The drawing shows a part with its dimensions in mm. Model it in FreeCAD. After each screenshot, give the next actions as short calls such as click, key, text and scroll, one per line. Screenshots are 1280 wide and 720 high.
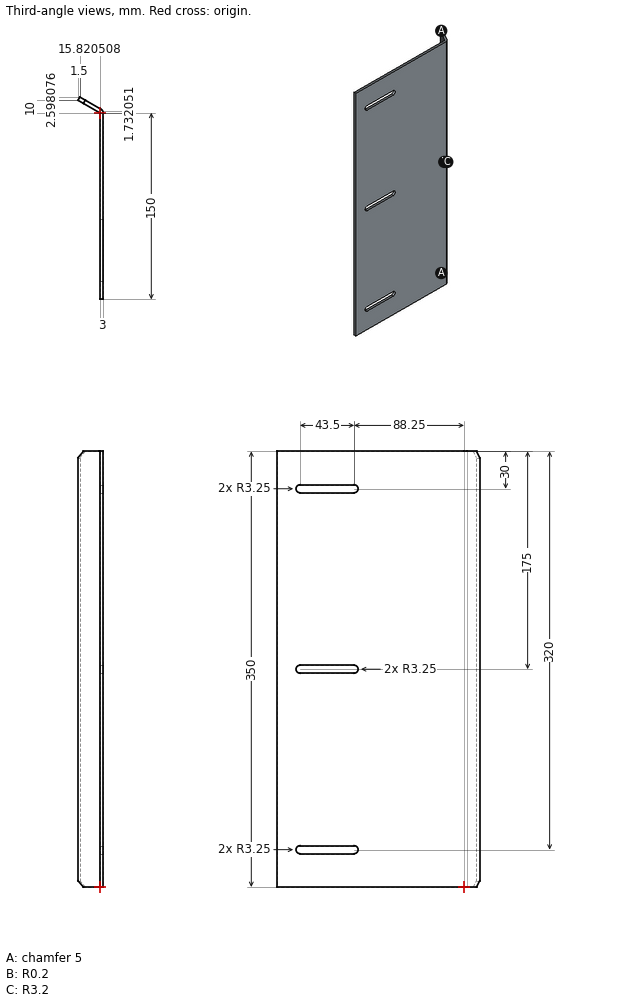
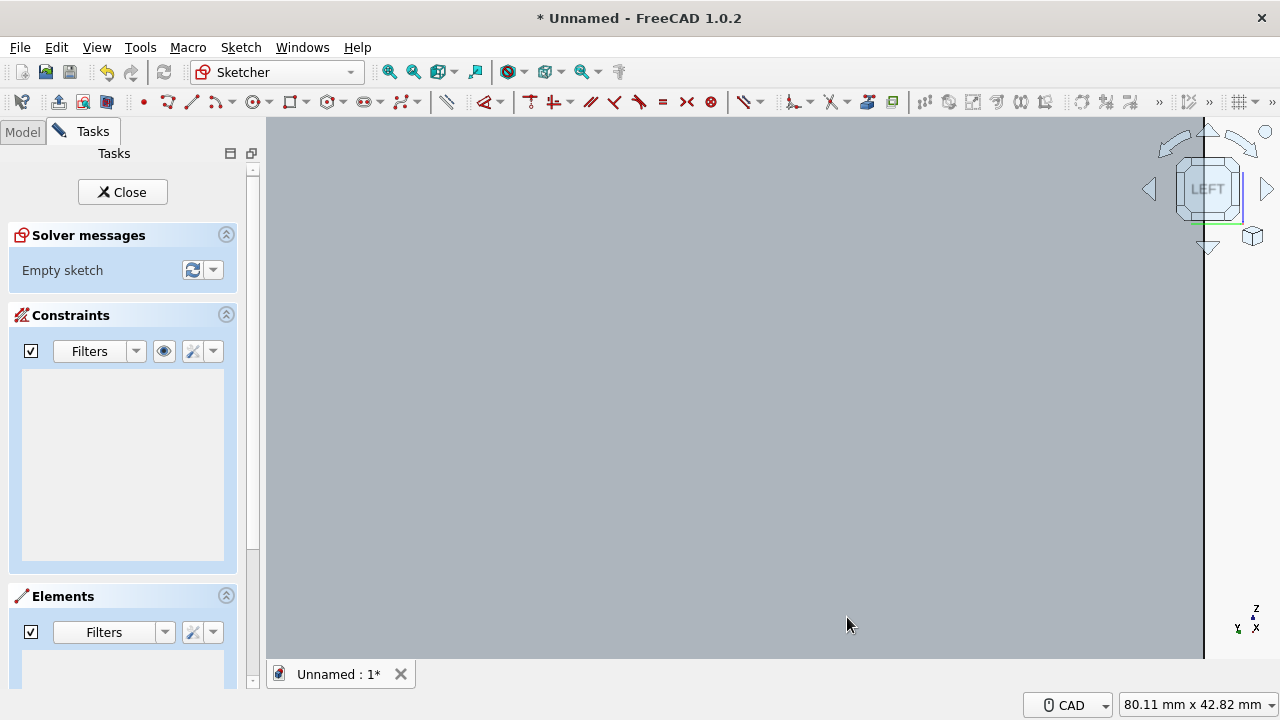
key(g)
key(s)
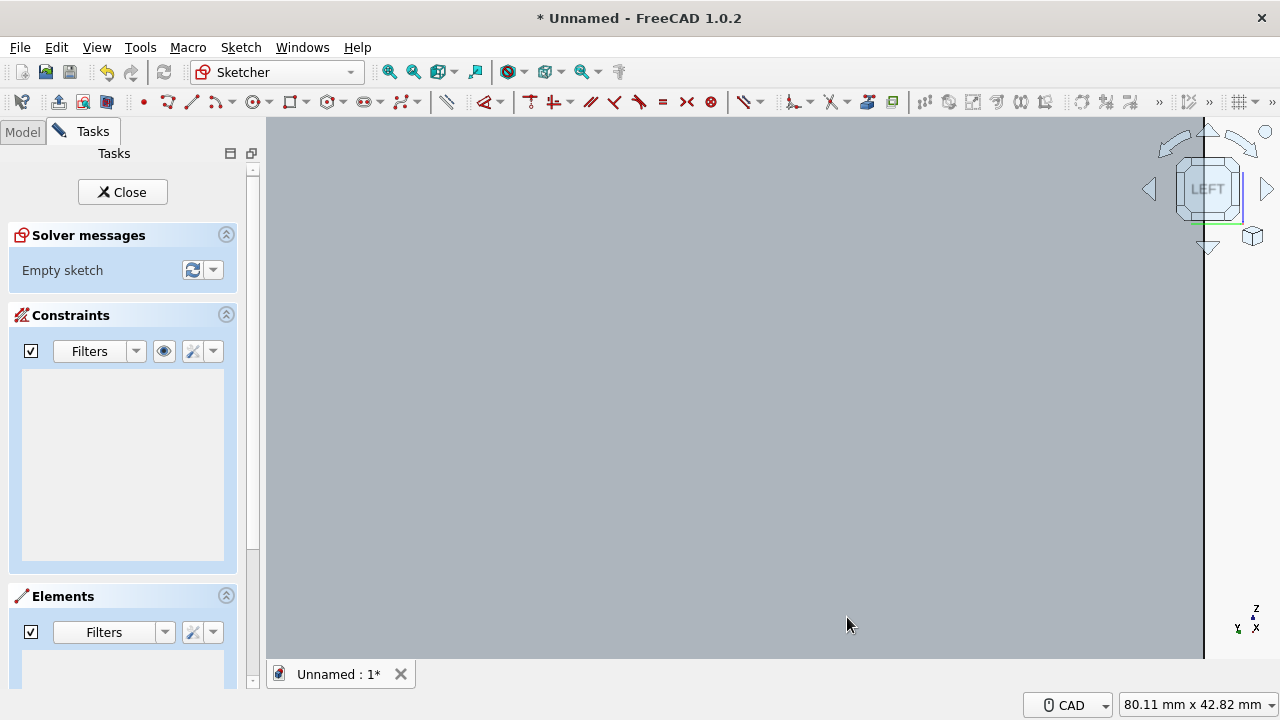
click(422, 378)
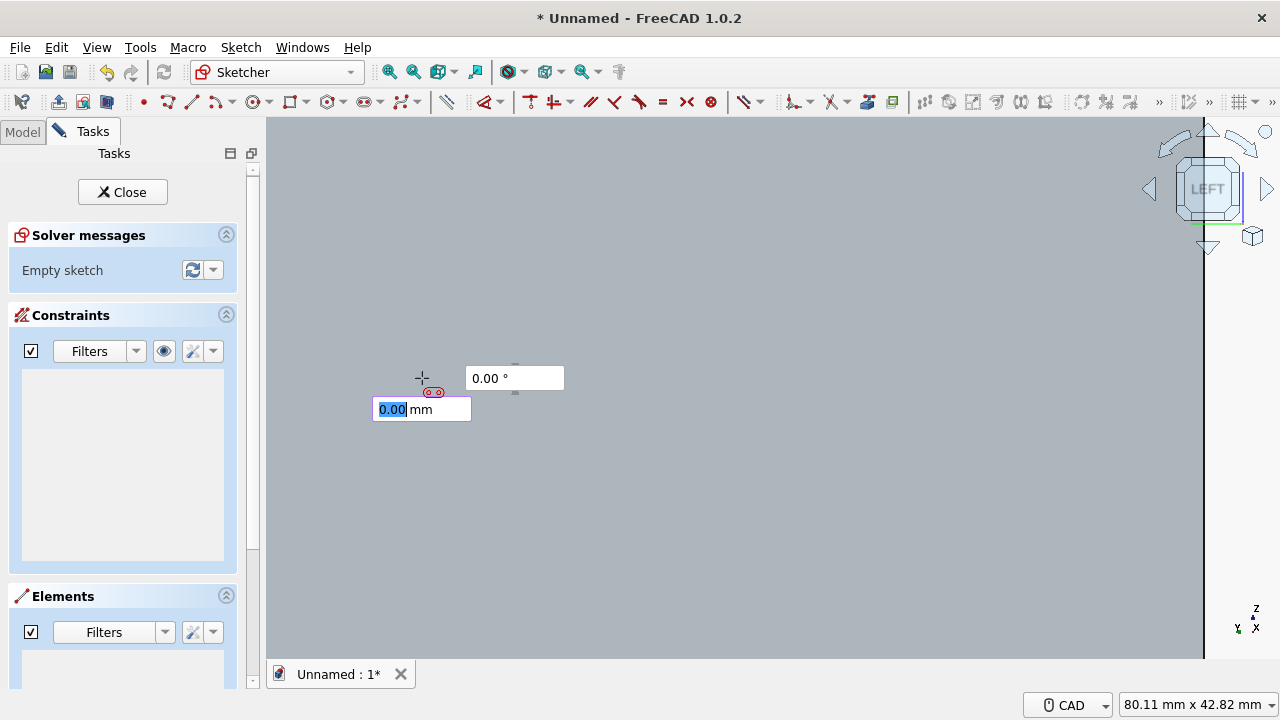
click(973, 378)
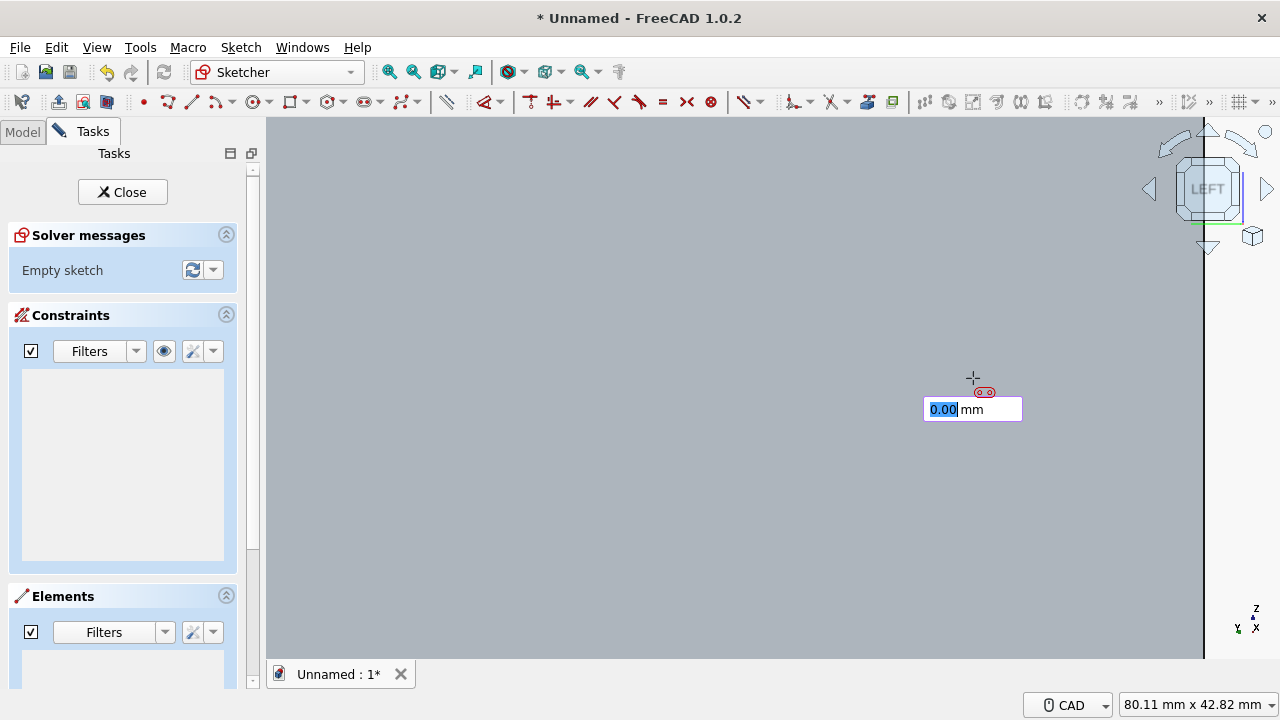
click(697, 419)
key(Escape)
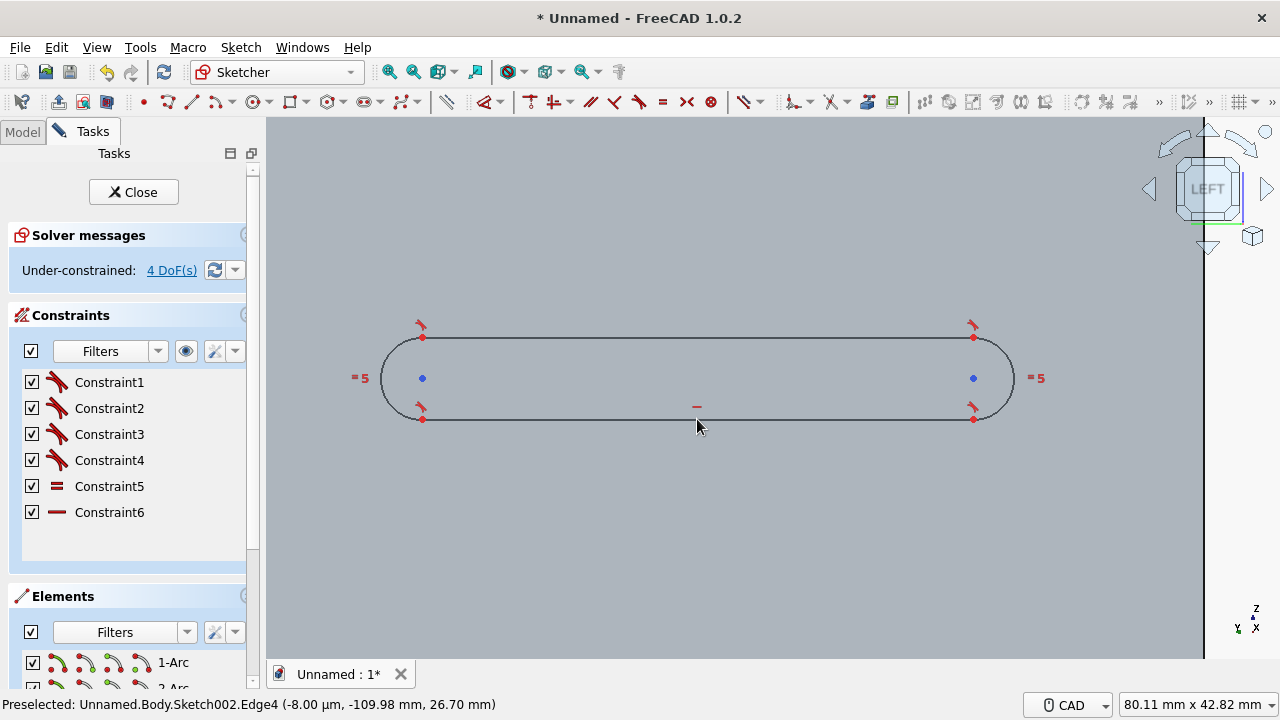
click(484, 102)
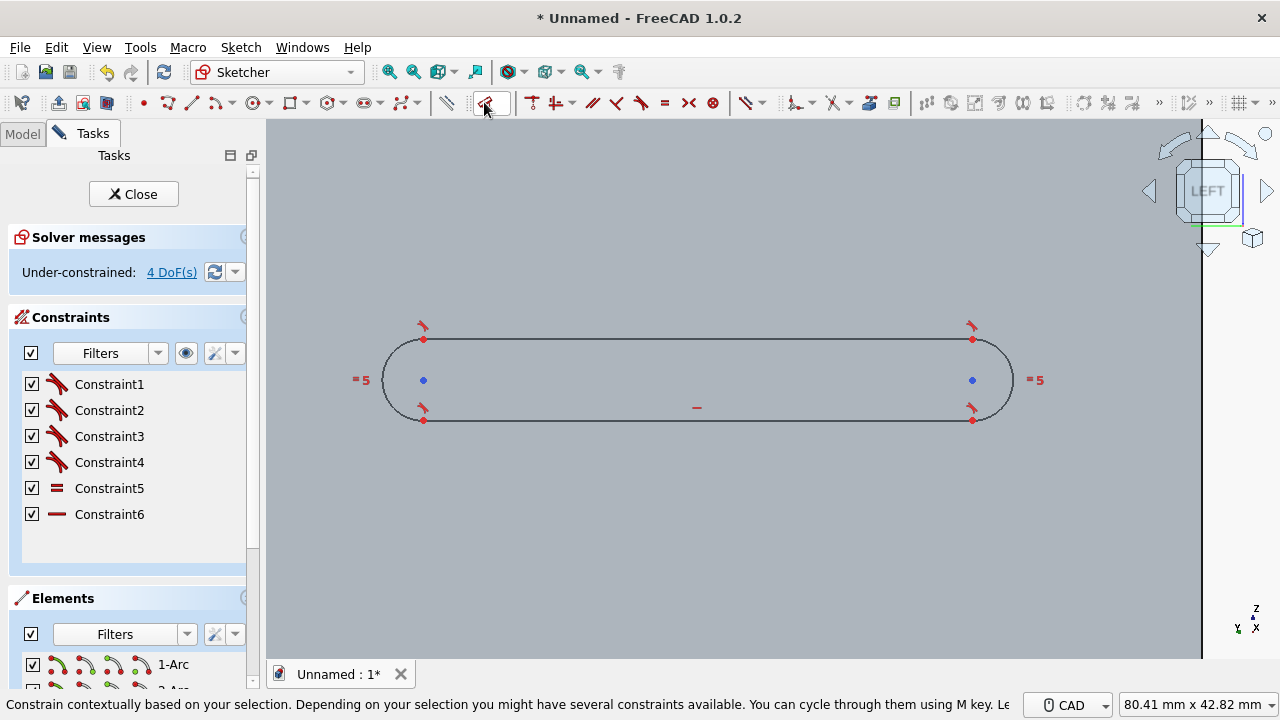
click(390, 356)
click(364, 337)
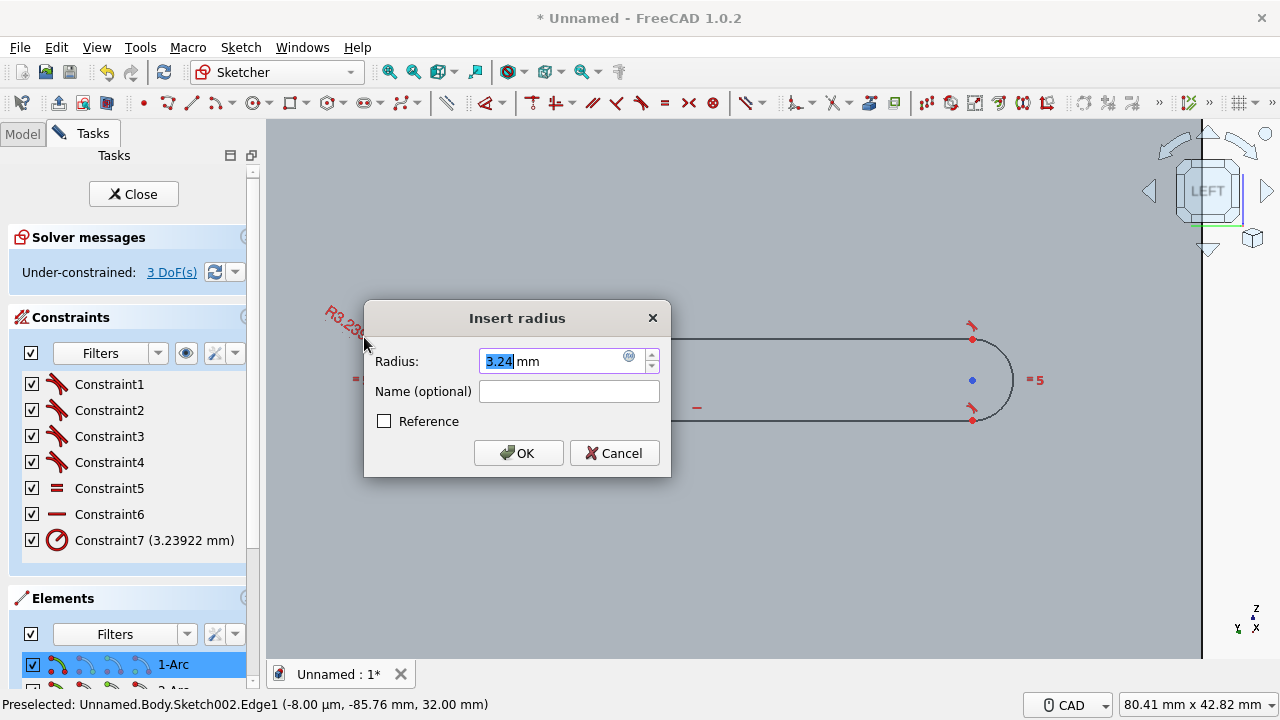
text(3.25)
key(Return)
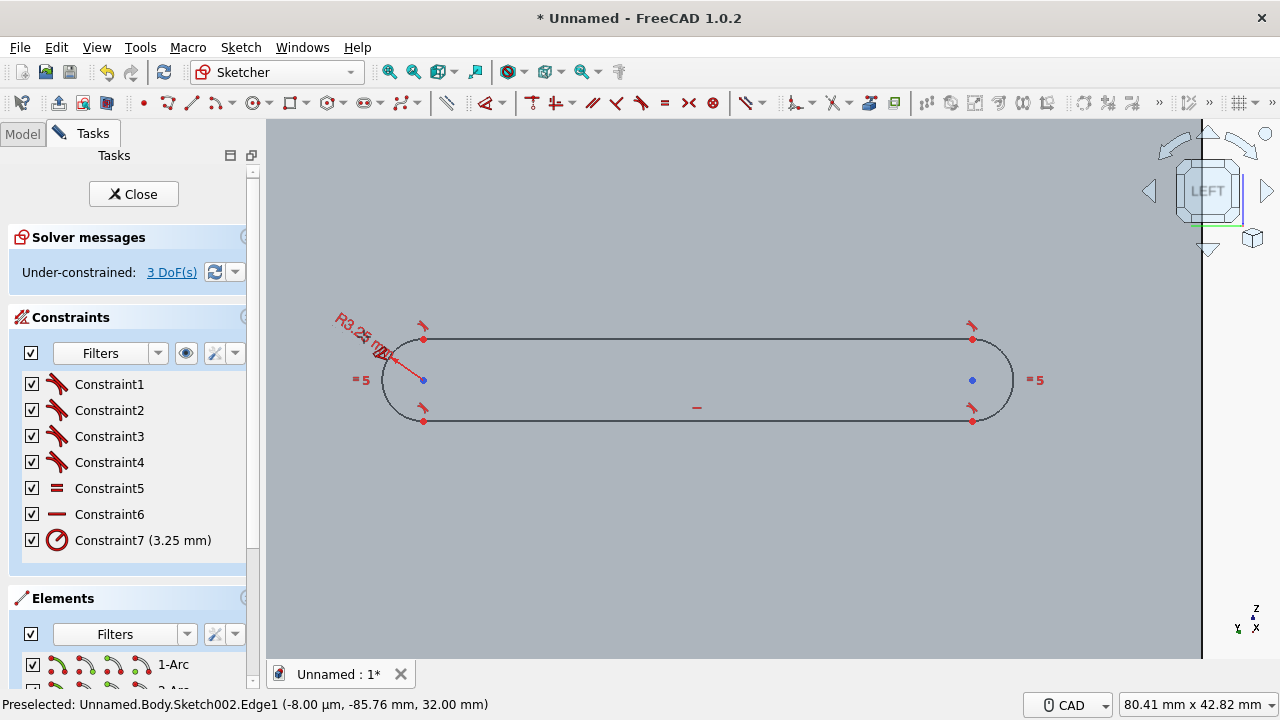
click(588, 339)
click(698, 305)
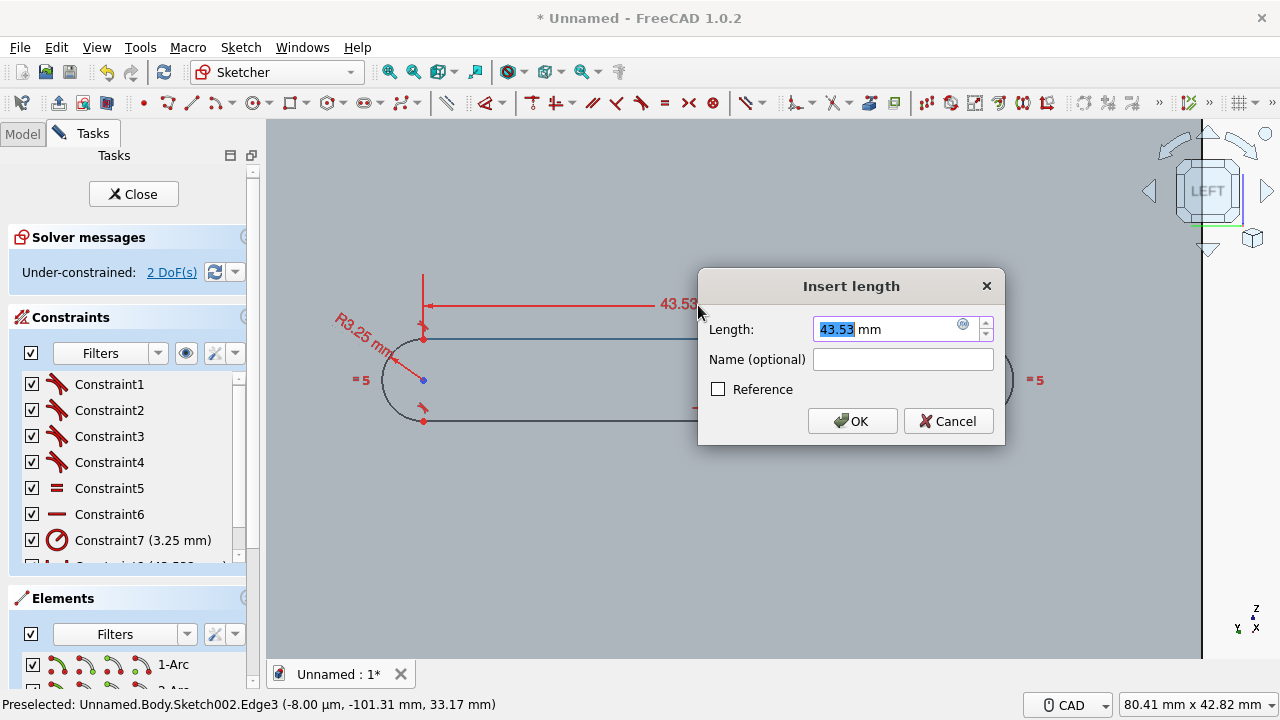
text(43.5)
key(Return)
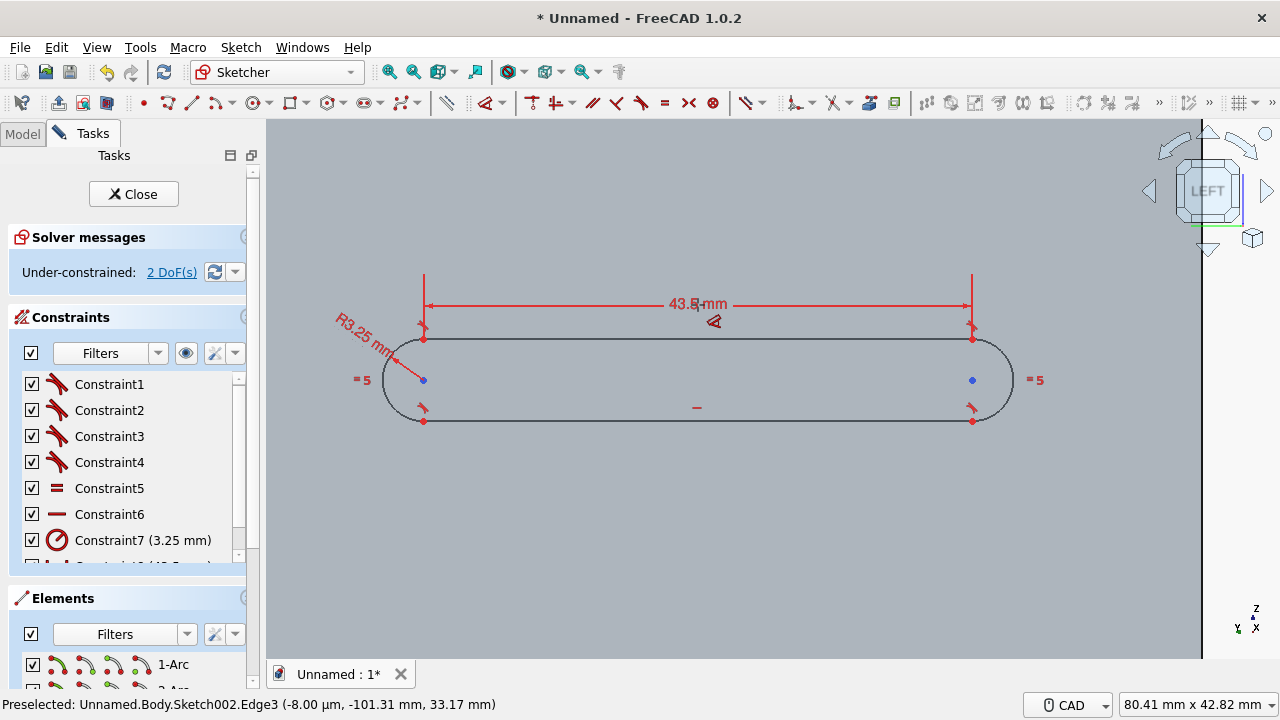
click(424, 380)
click(458, 264)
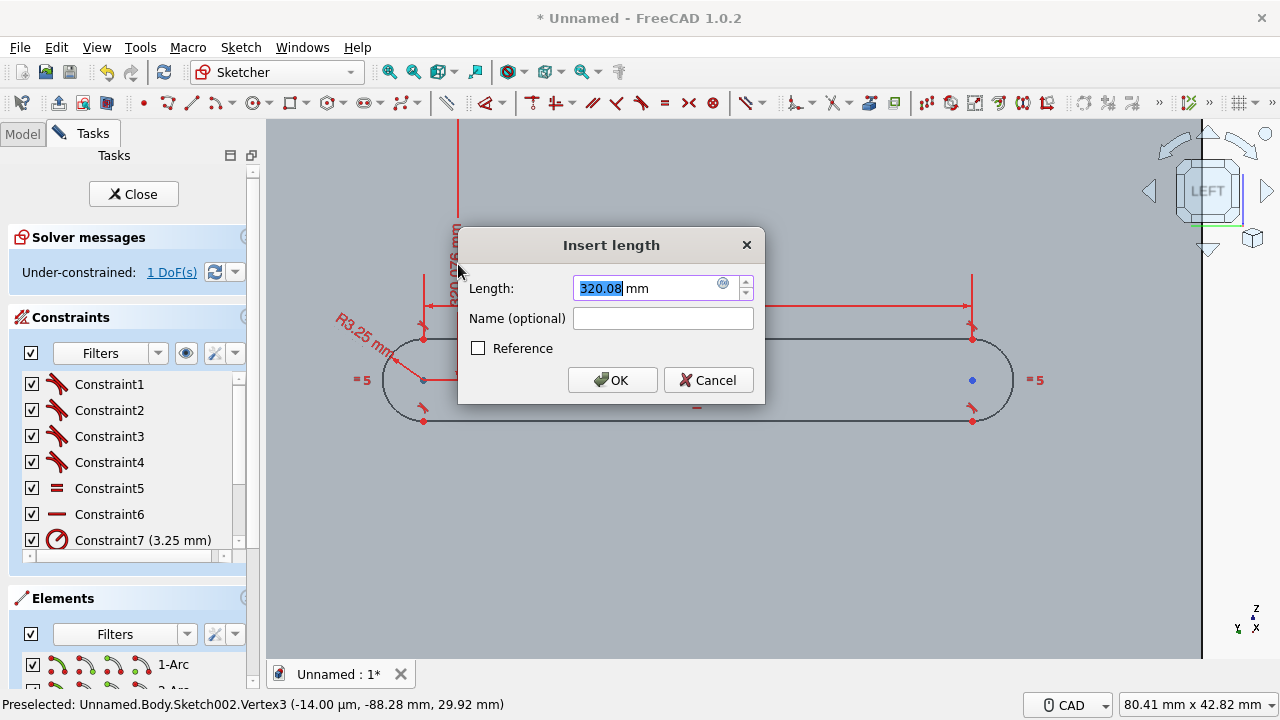
text(320)
key(Return)